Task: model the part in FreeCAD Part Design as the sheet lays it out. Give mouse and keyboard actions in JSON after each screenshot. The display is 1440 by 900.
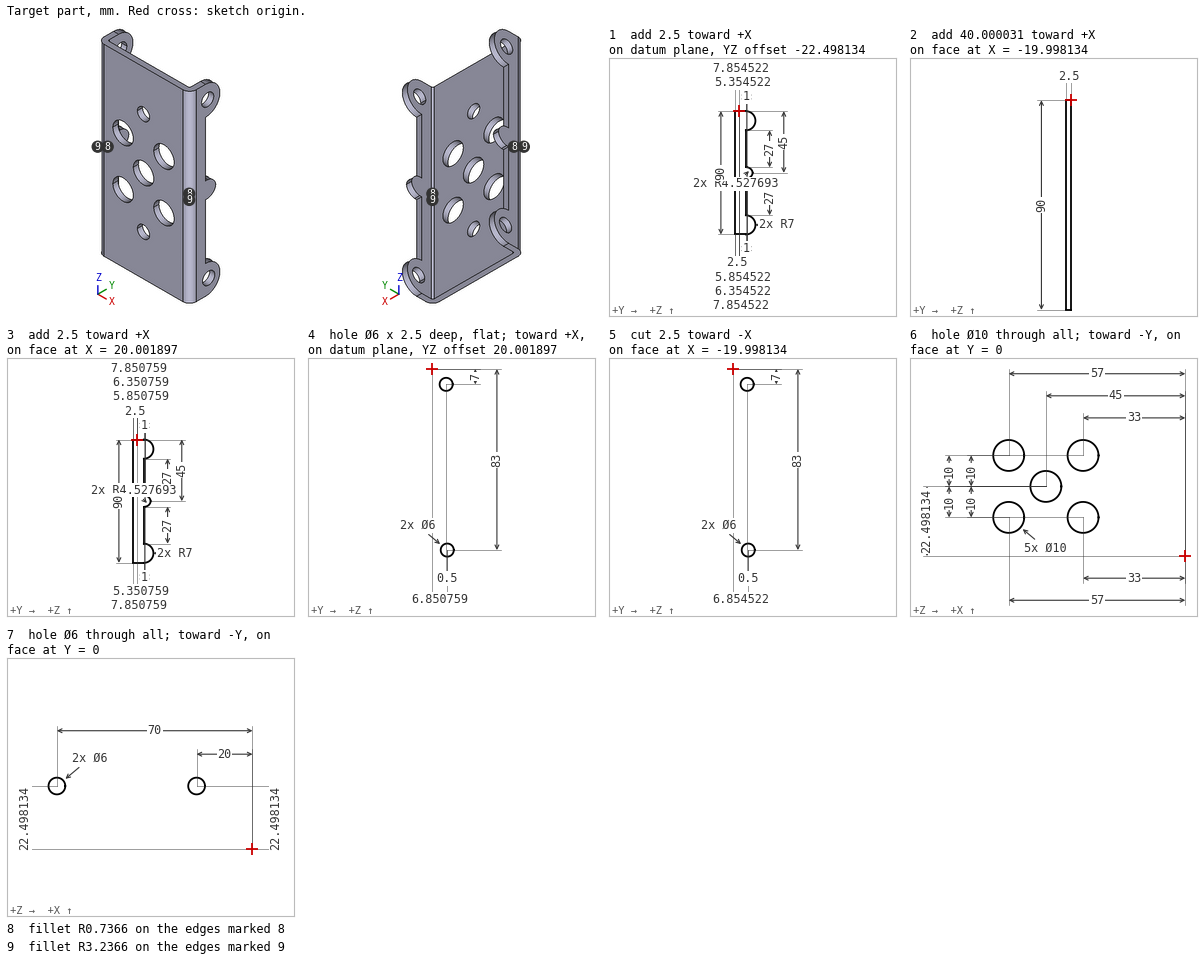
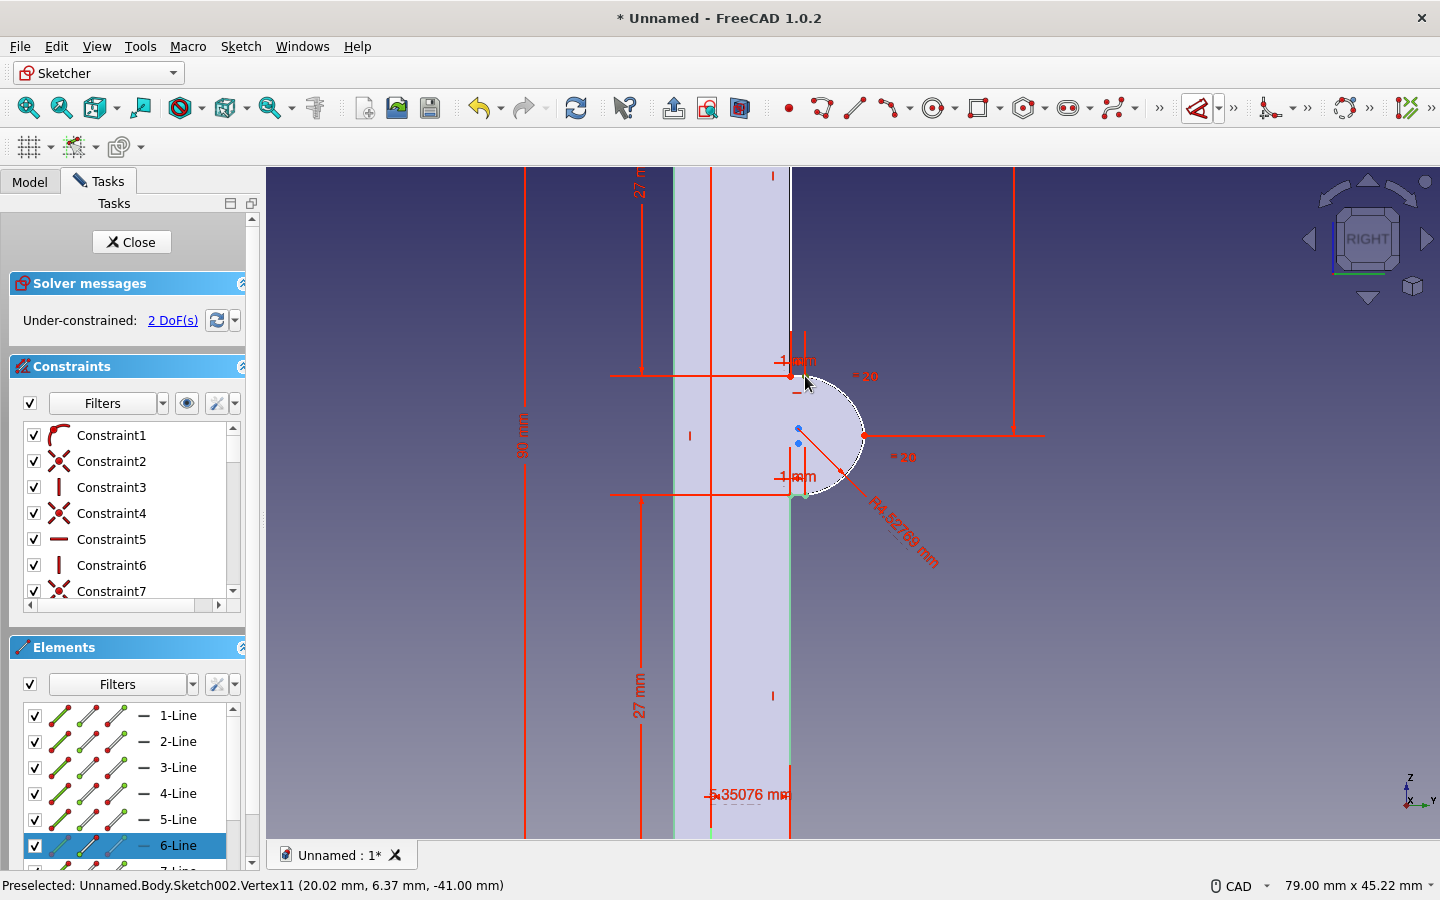
{"action": "key", "text": "l"}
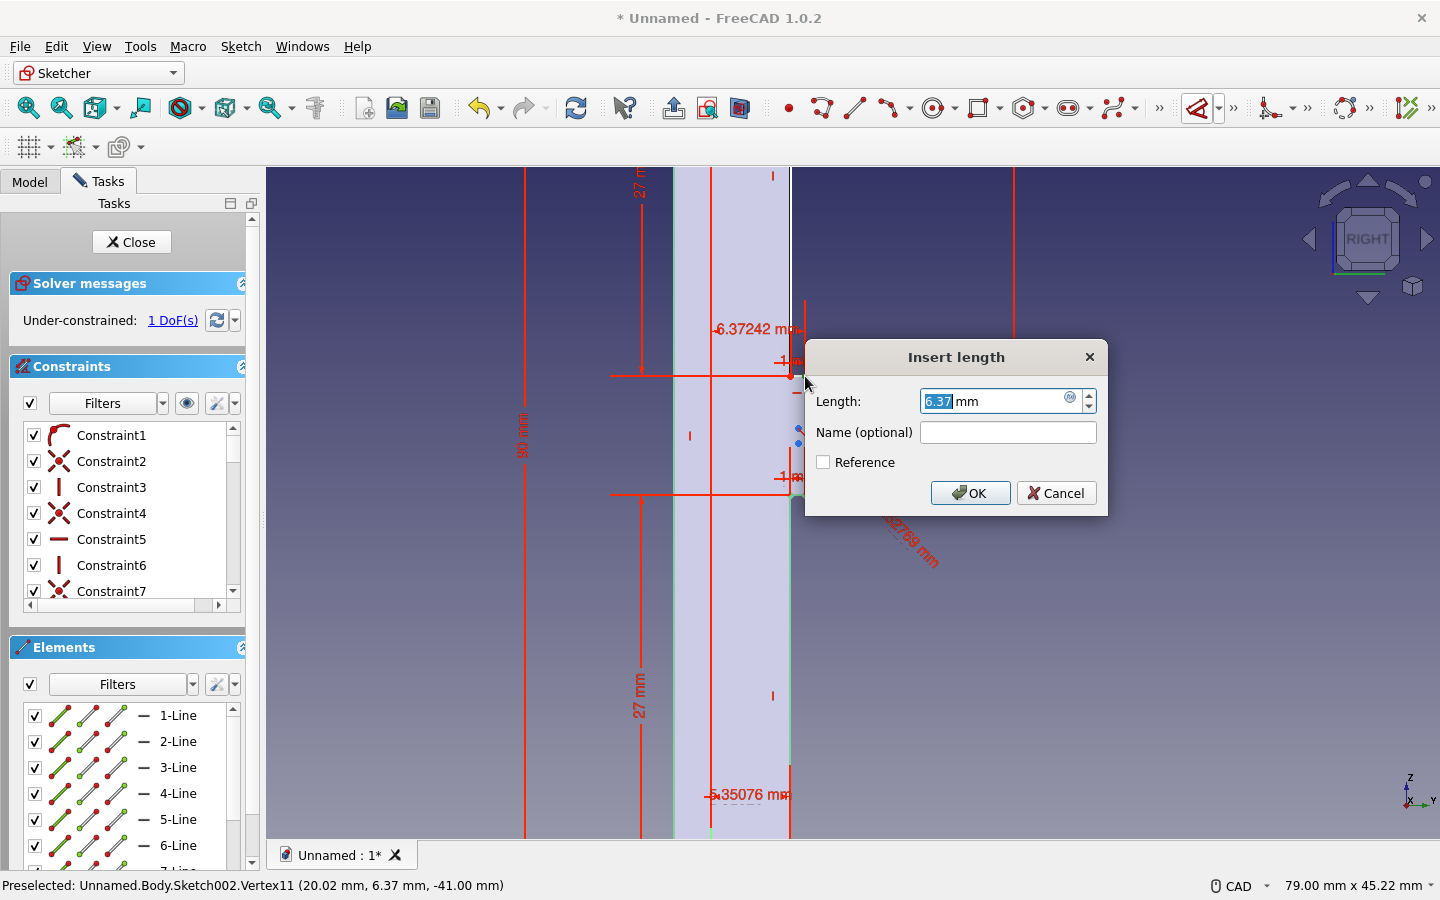
{"action": "type", "text": "6.350759"}
{"action": "key", "text": "Return"}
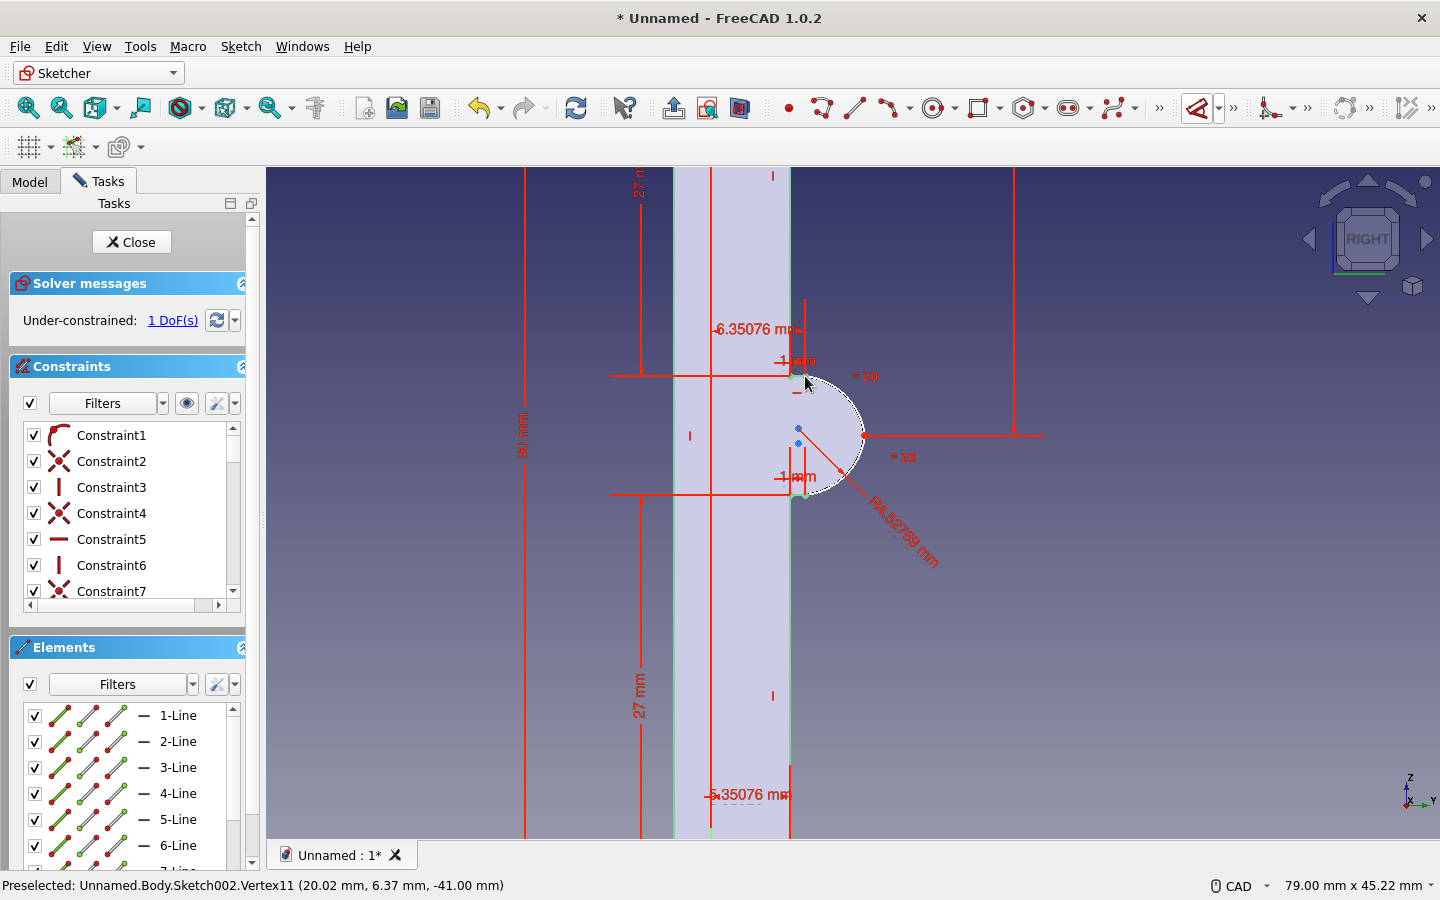
{"action": "left_click", "coordinate": [798, 428]}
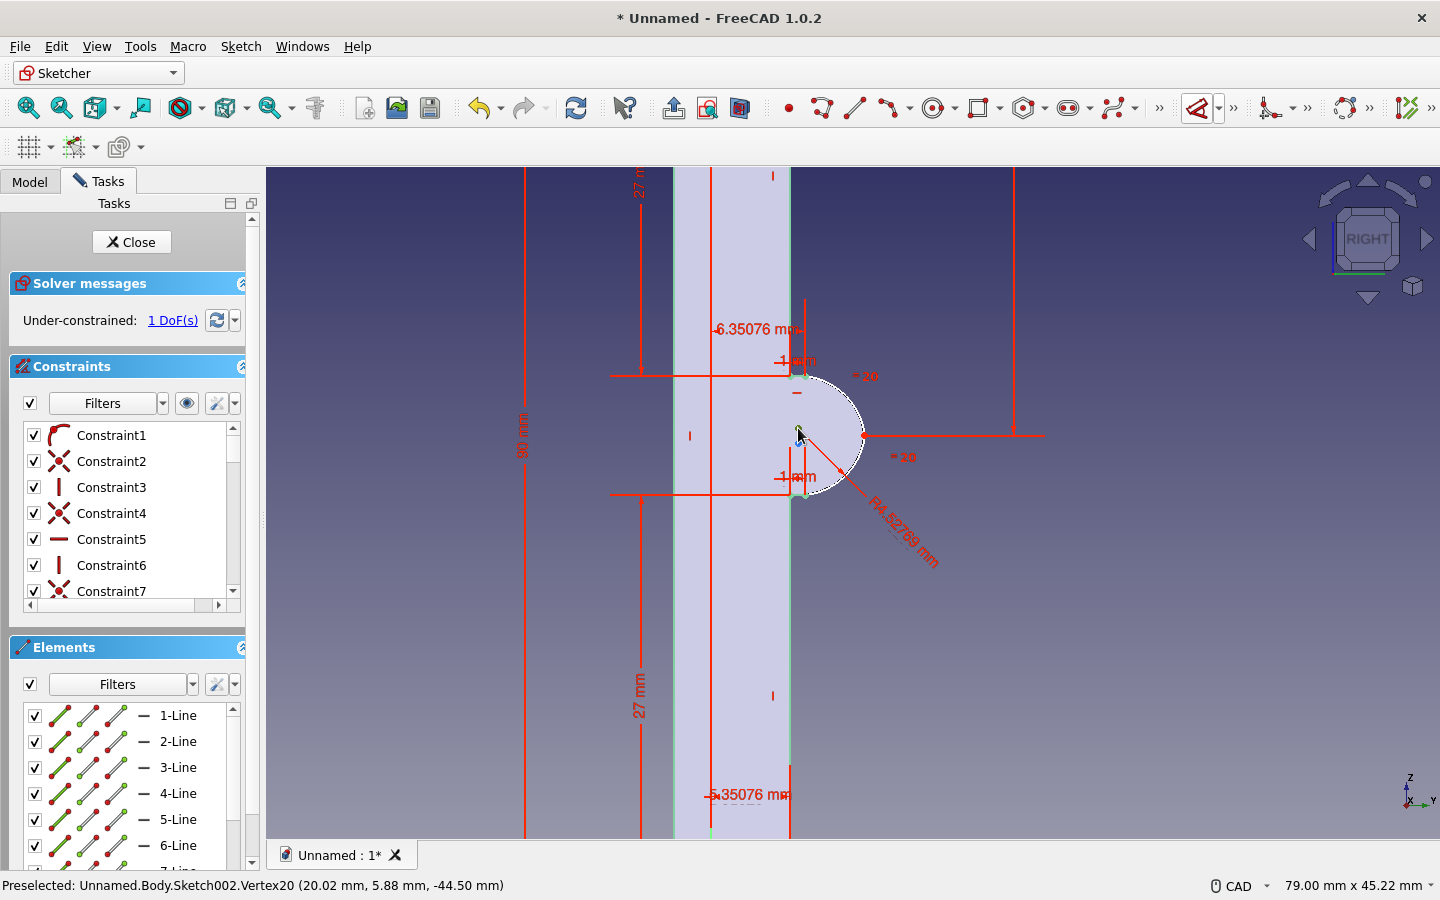
{"action": "key", "text": "l"}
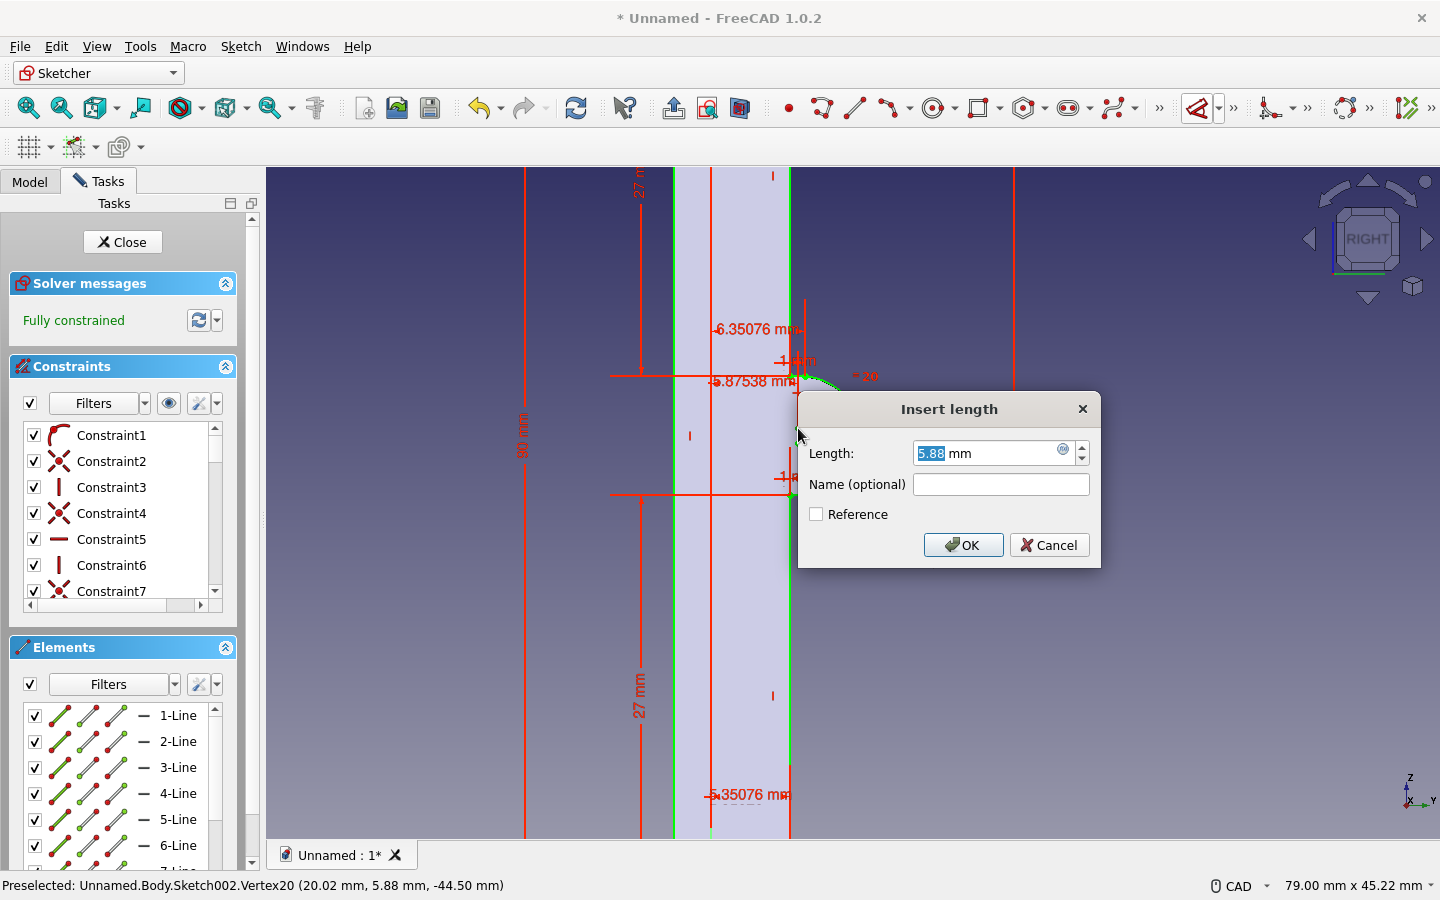
{"action": "type", "text": "5.850759"}
{"action": "key", "text": "Return"}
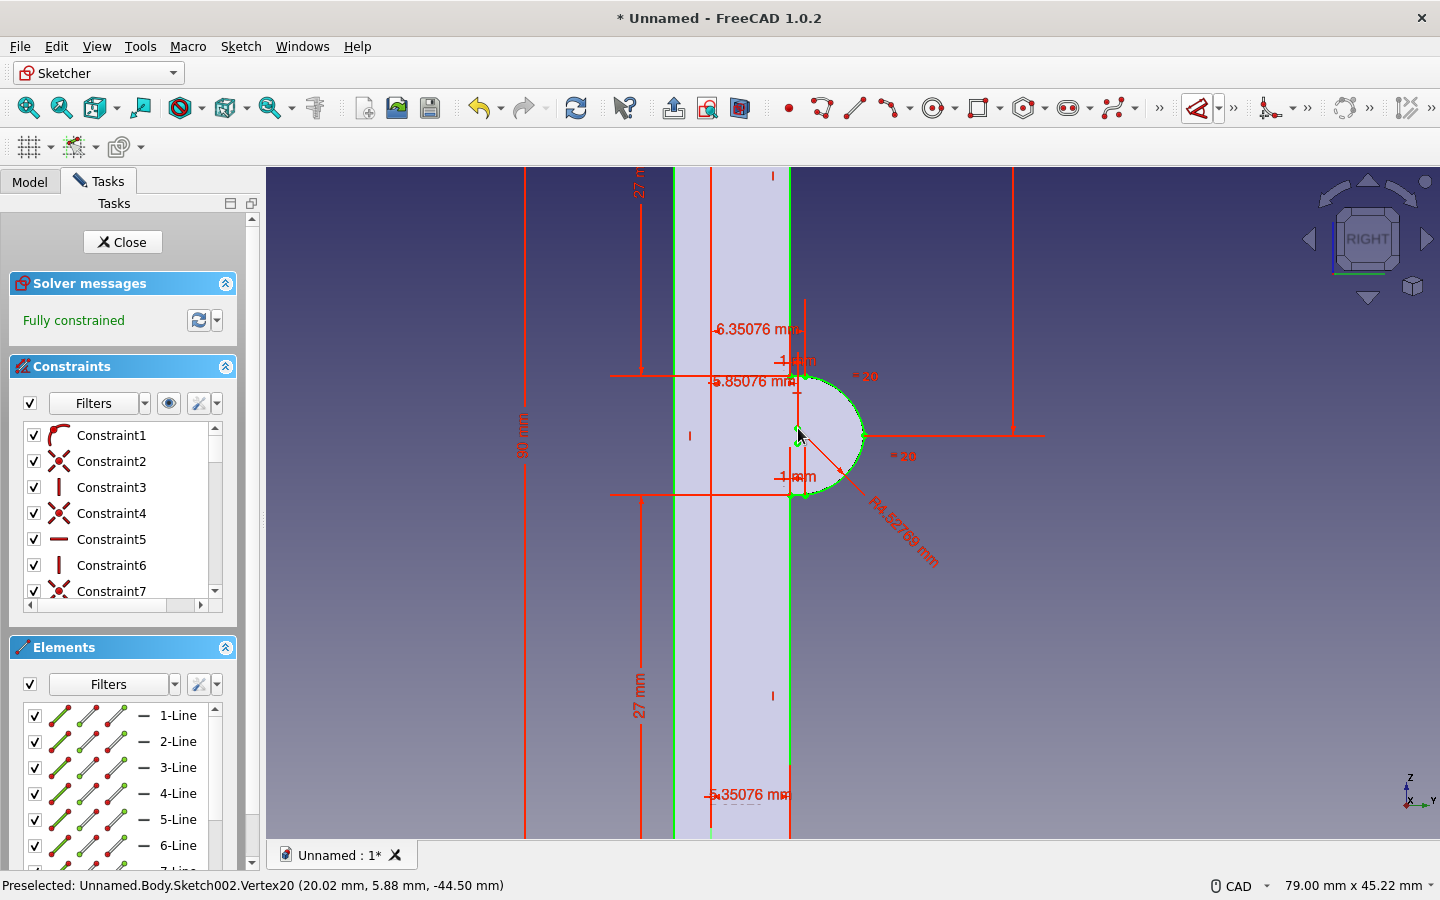
{"action": "left_click", "coordinate": [123, 242]}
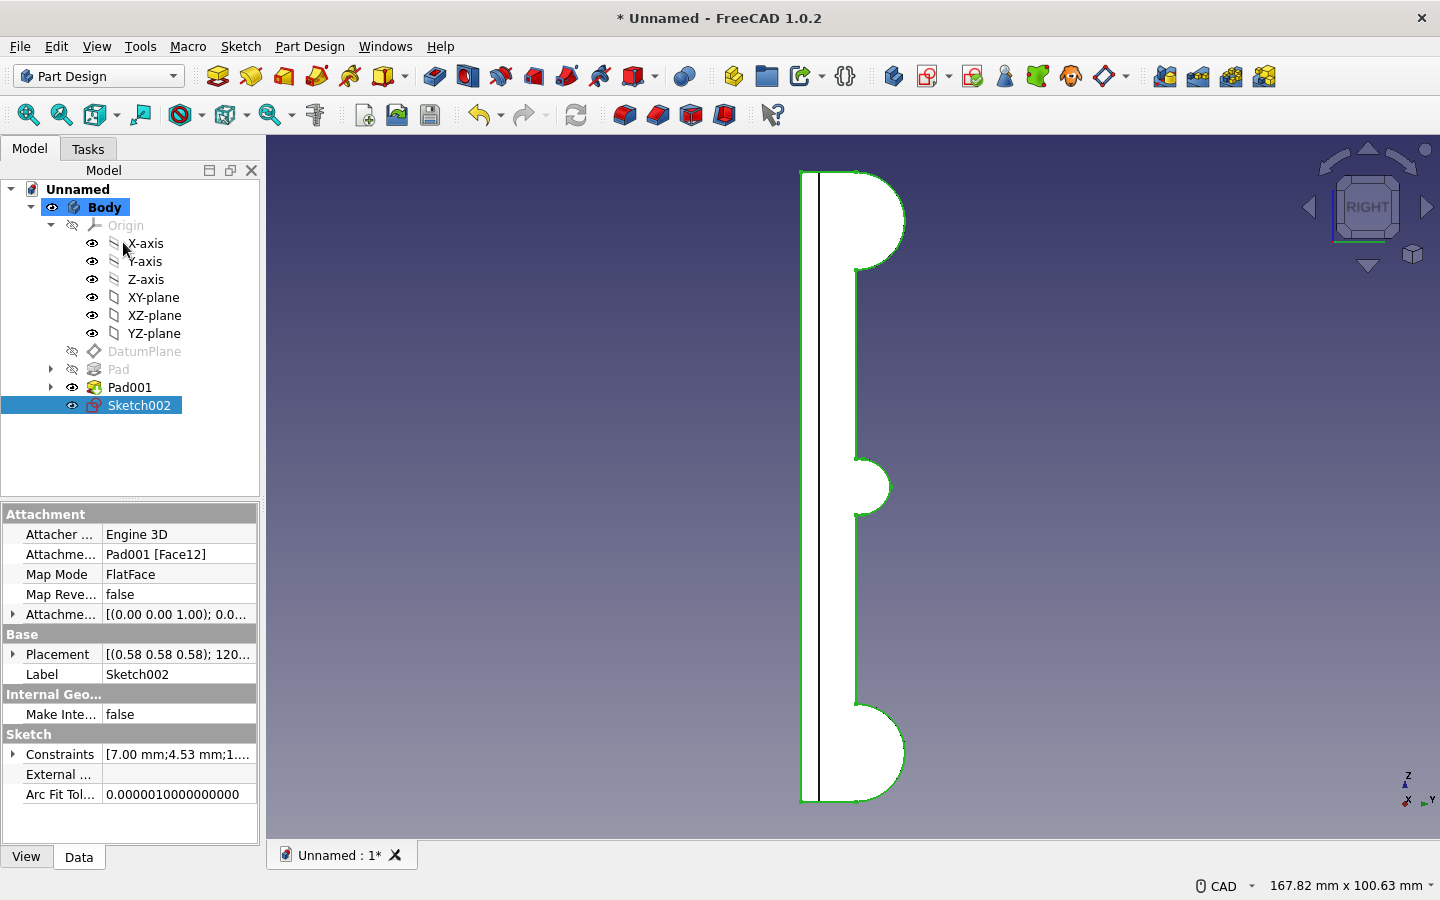
{"action": "left_click", "coordinate": [218, 76]}